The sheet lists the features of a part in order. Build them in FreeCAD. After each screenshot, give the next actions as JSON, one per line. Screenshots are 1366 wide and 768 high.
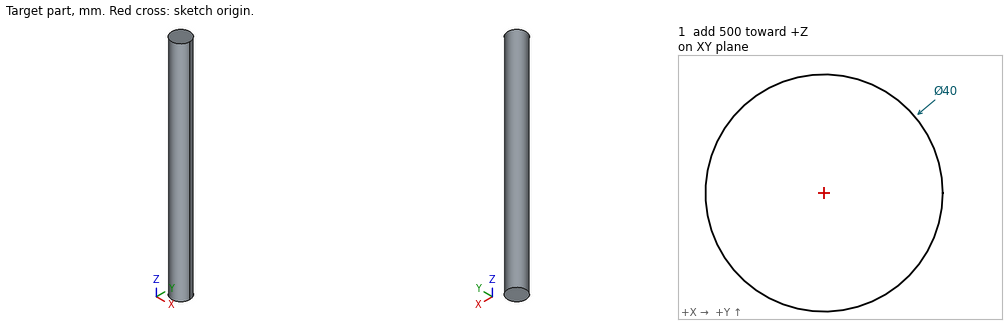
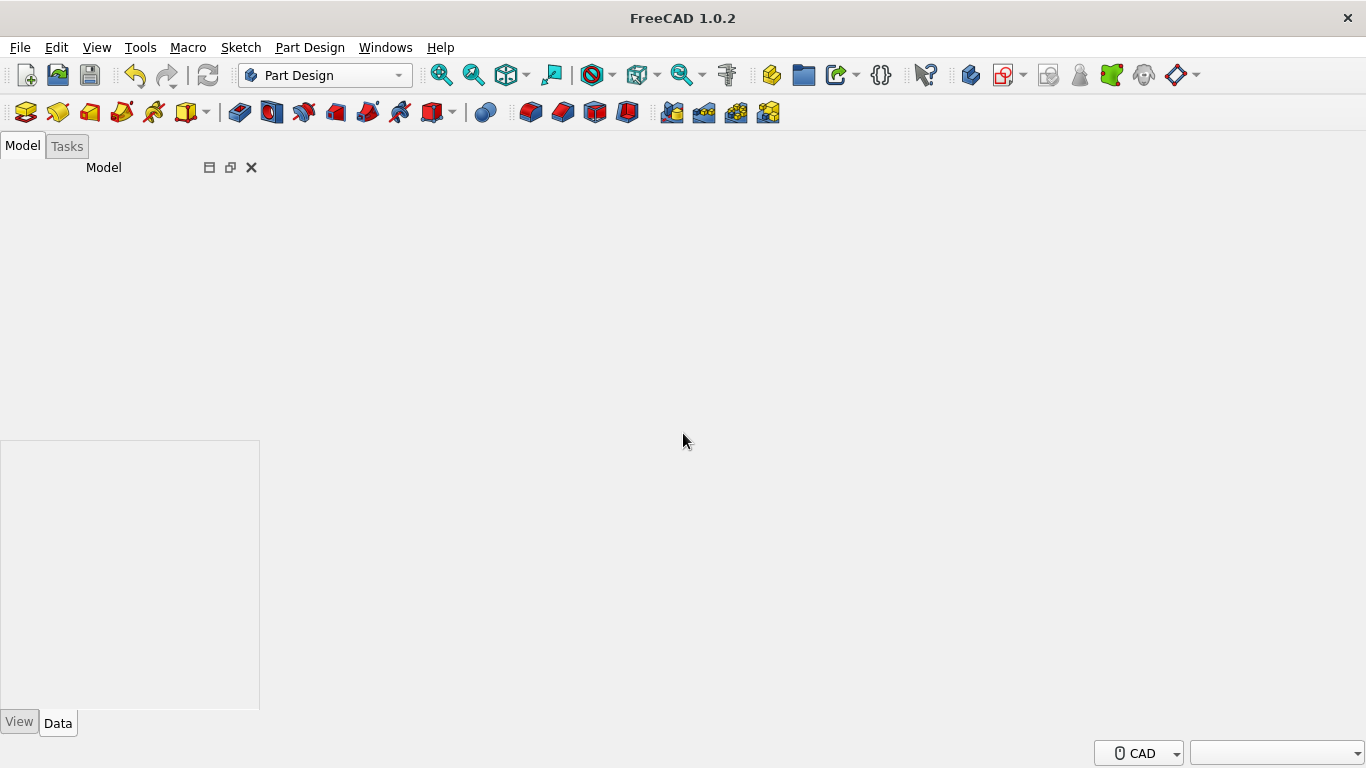
{"action": "left_click", "coordinate": [26, 76]}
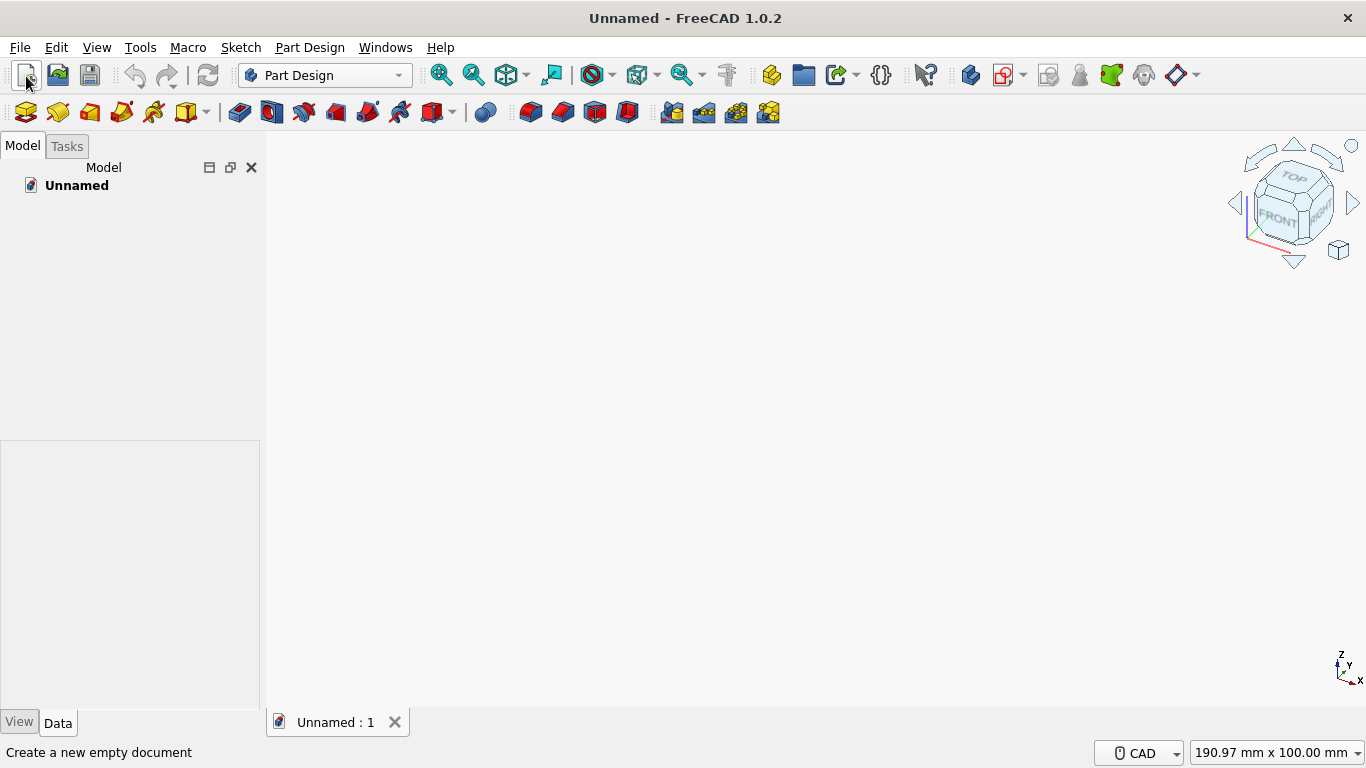
{"action": "left_click", "coordinate": [1004, 76]}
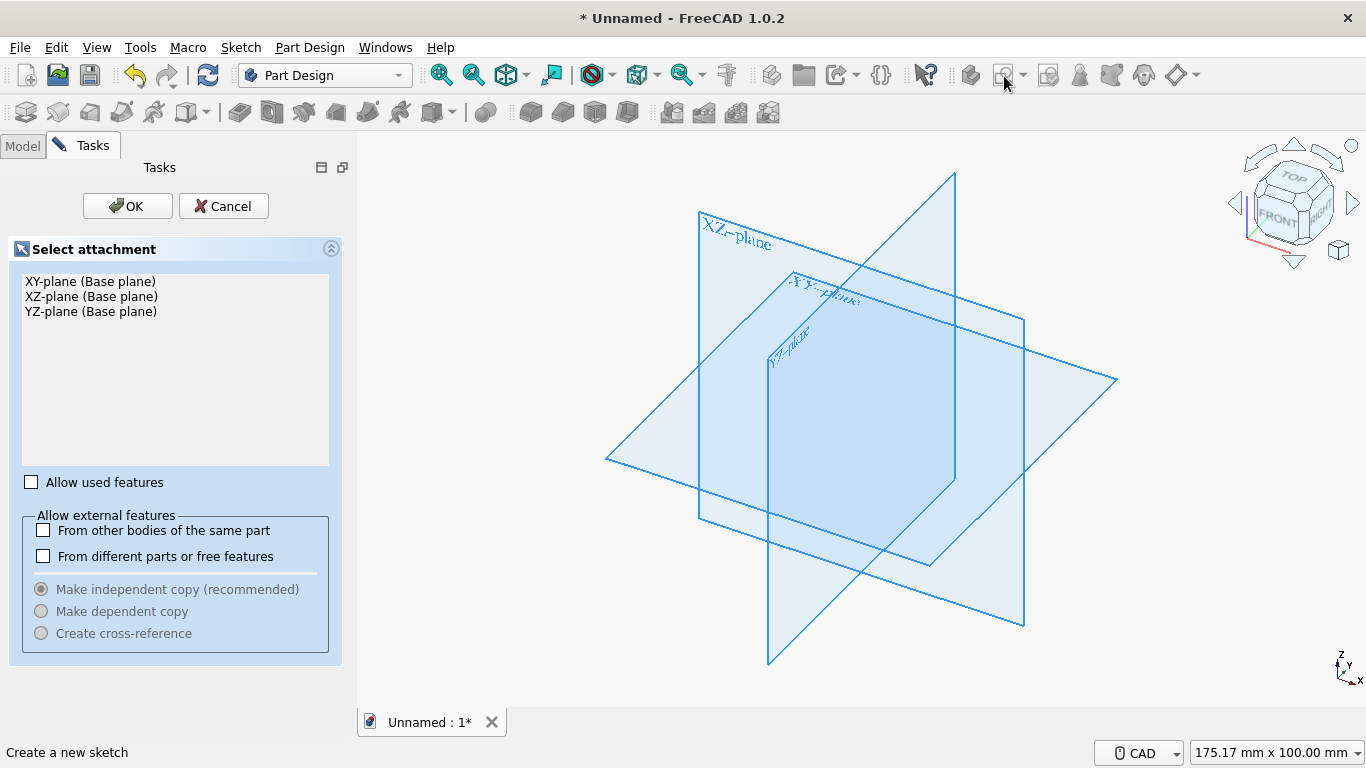
{"action": "left_click", "coordinate": [82, 282]}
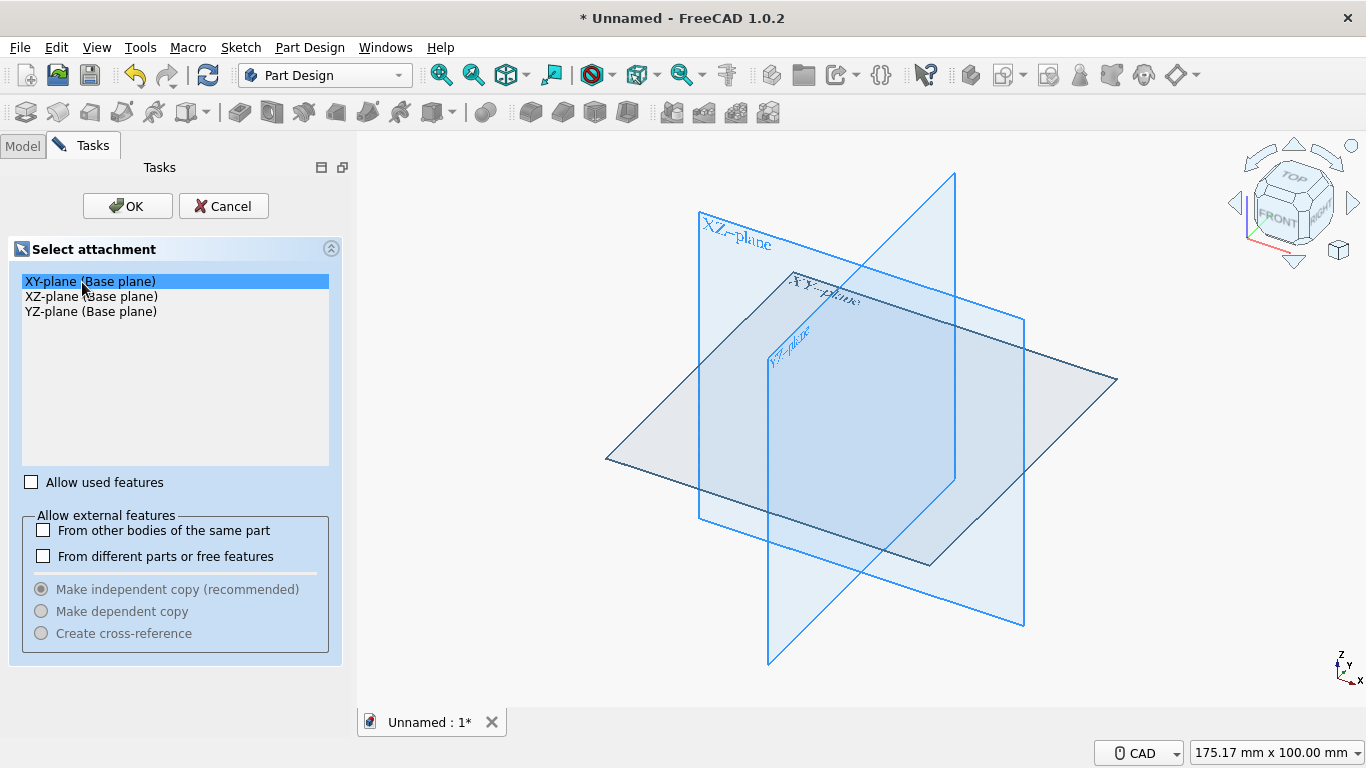
{"action": "left_click", "coordinate": [128, 206]}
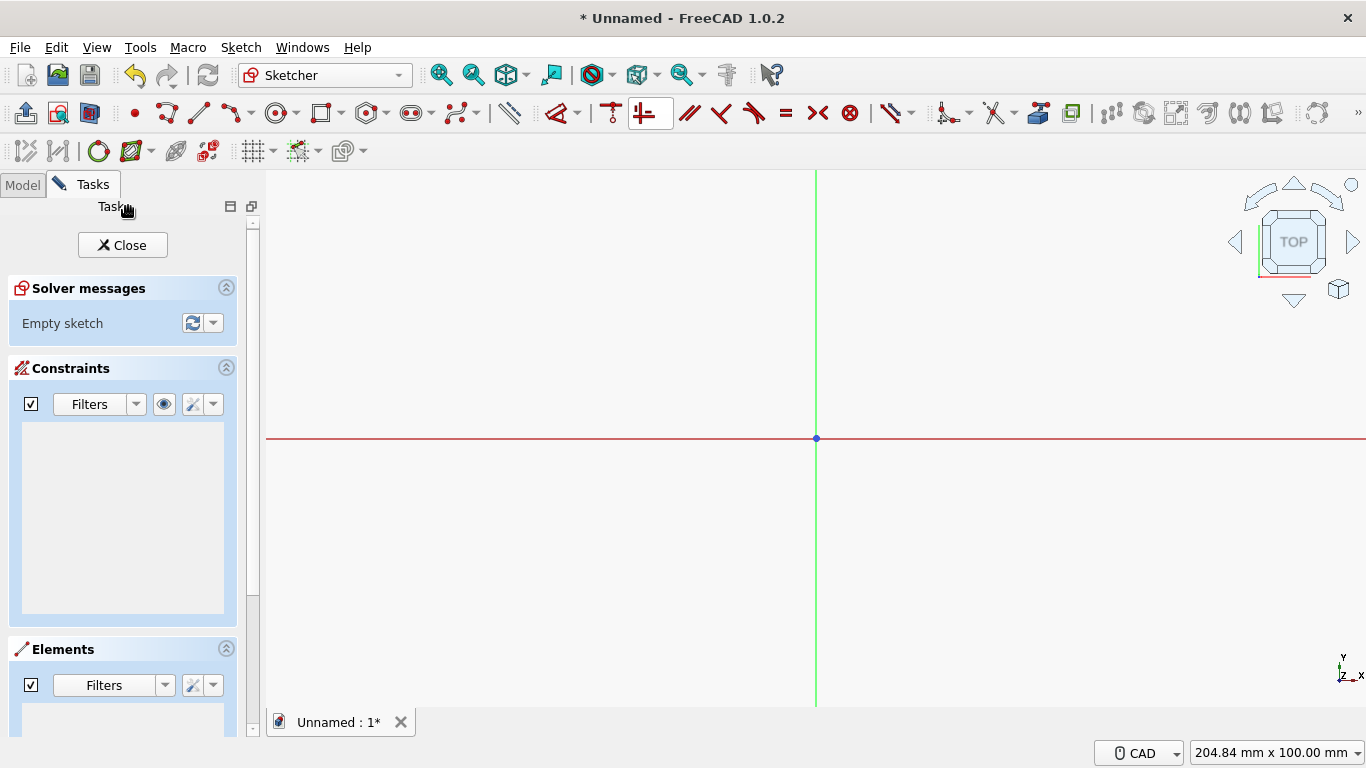
{"action": "scroll", "coordinate": [955, 439], "scroll_direction": "up", "scroll_amount": 2}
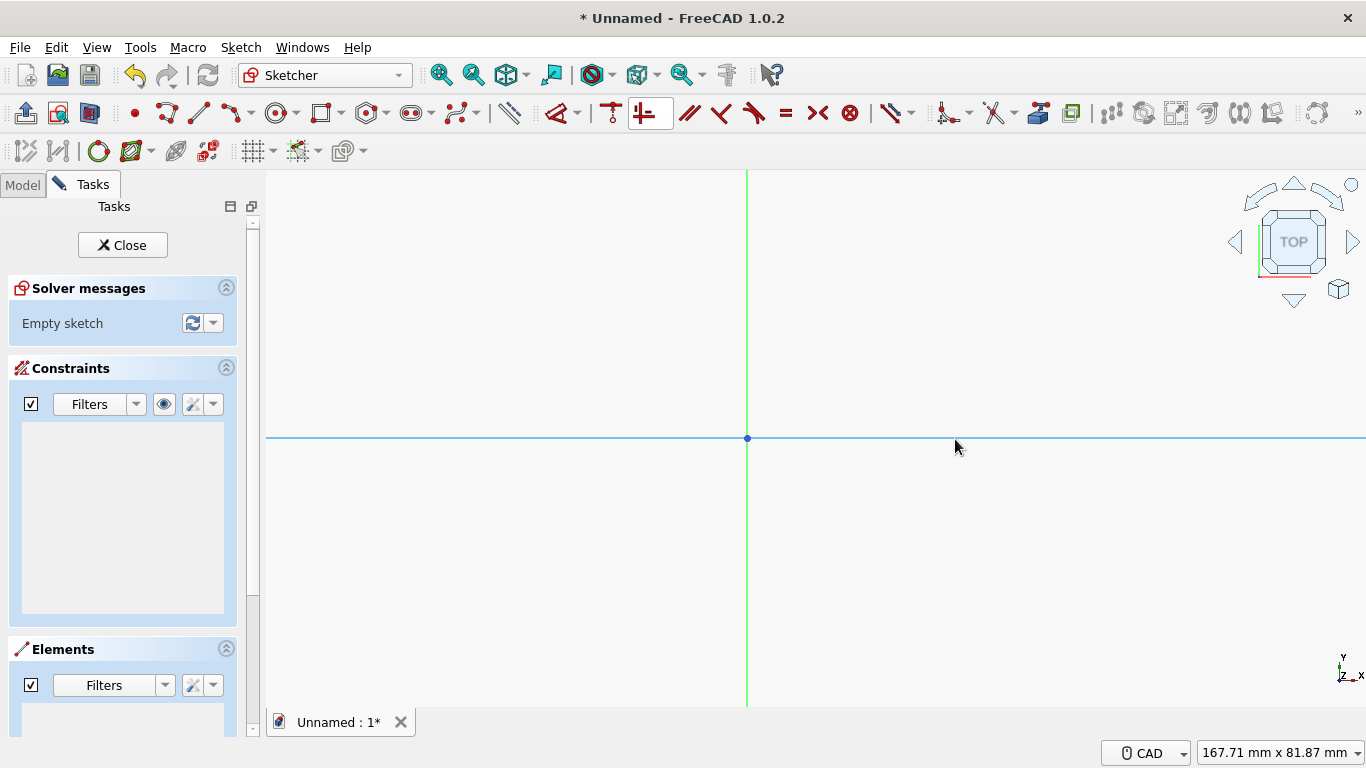
{"action": "left_click", "coordinate": [276, 114]}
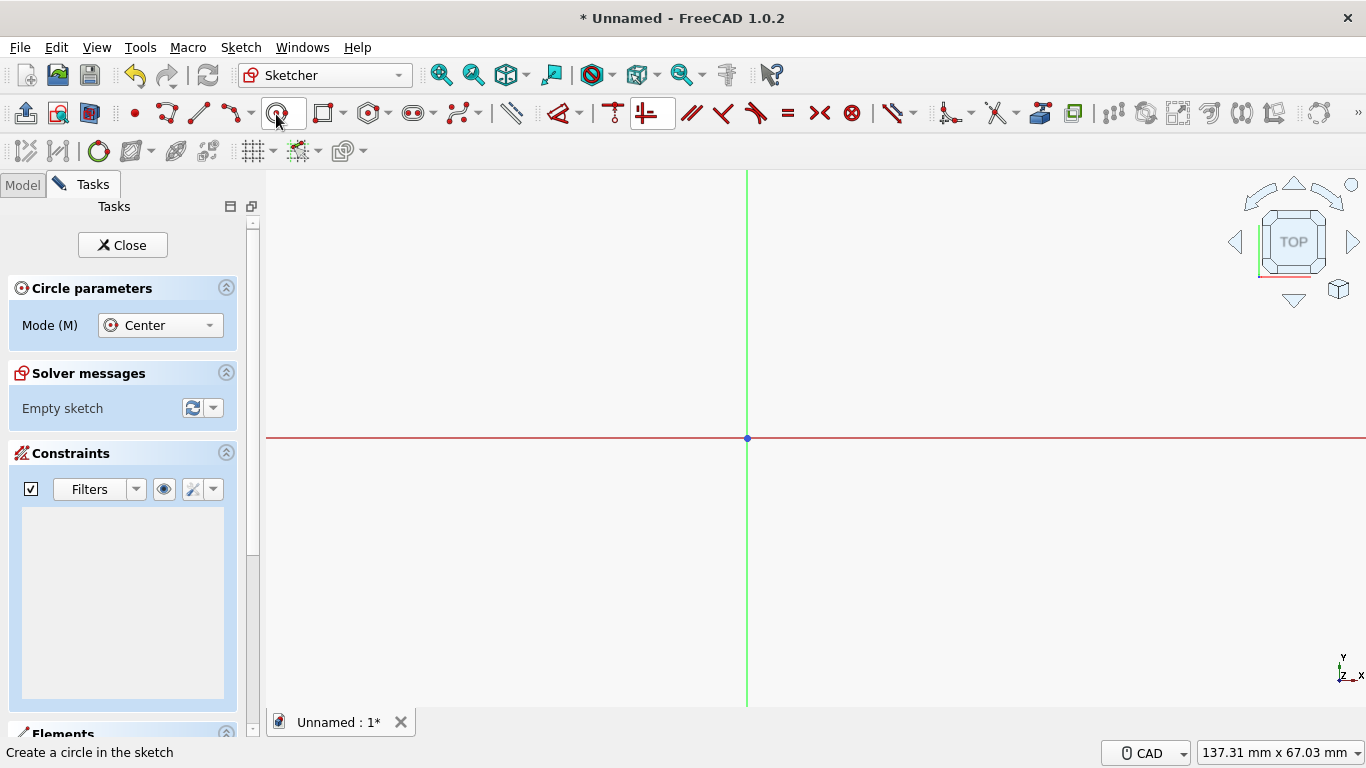
{"action": "left_click", "coordinate": [747, 438]}
{"action": "mouse_move", "coordinate": [861, 325]}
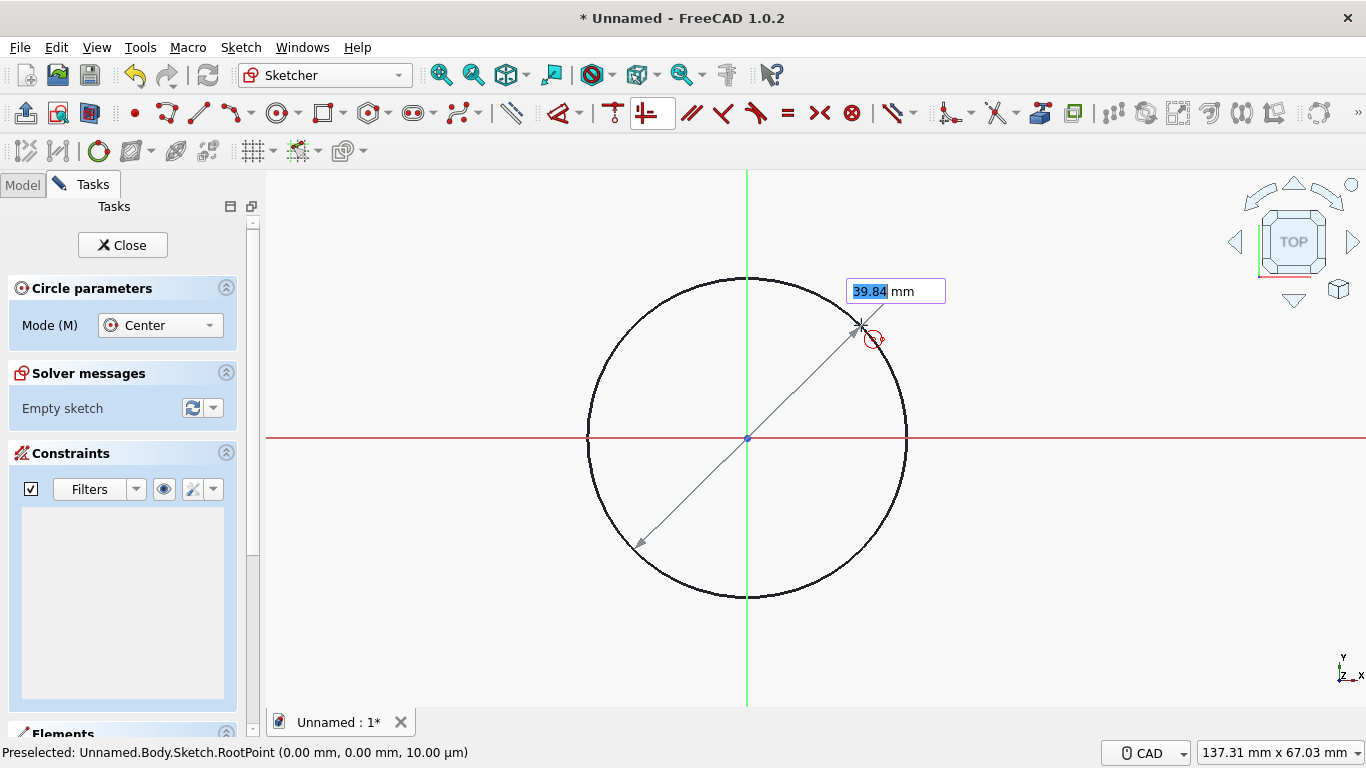
{"action": "type", "text": "40"}
{"action": "key", "text": "Return"}
{"action": "key", "text": "Escape"}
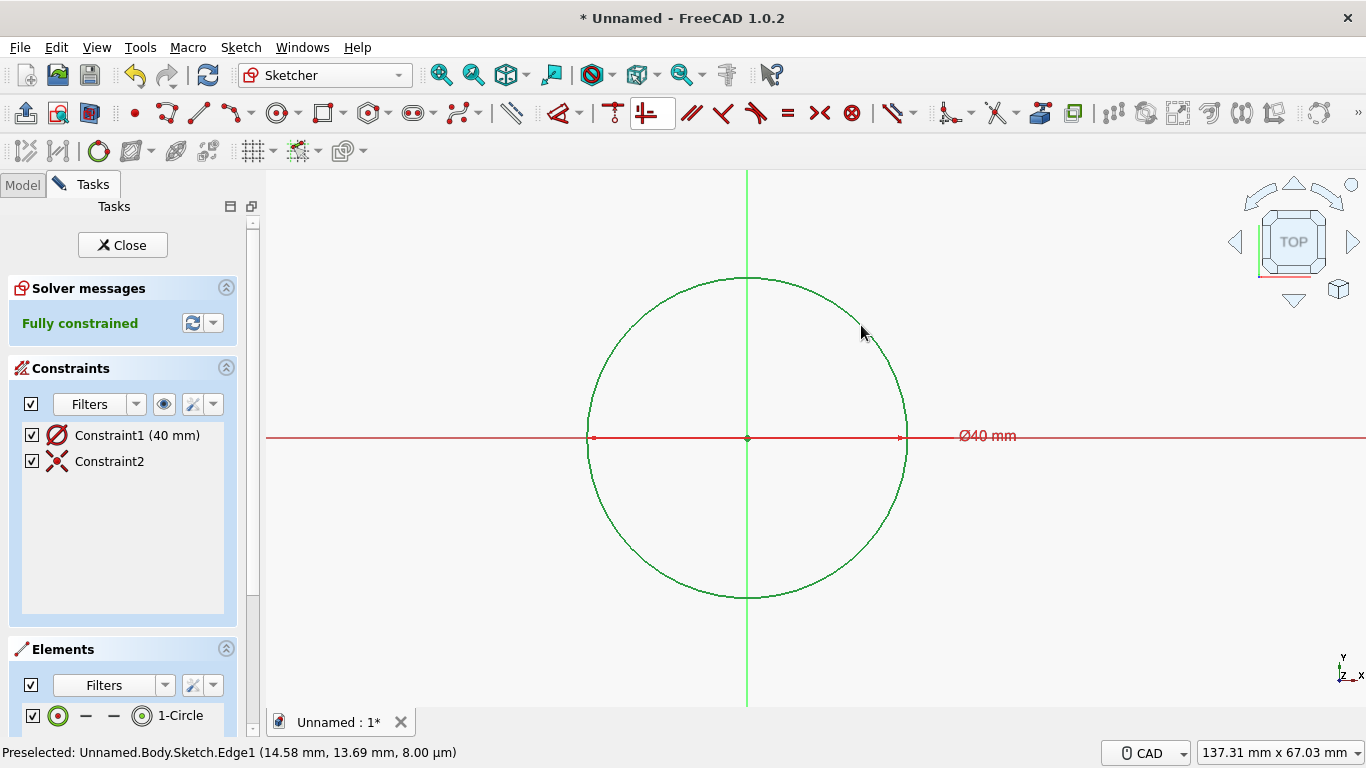
{"action": "left_click", "coordinate": [123, 245]}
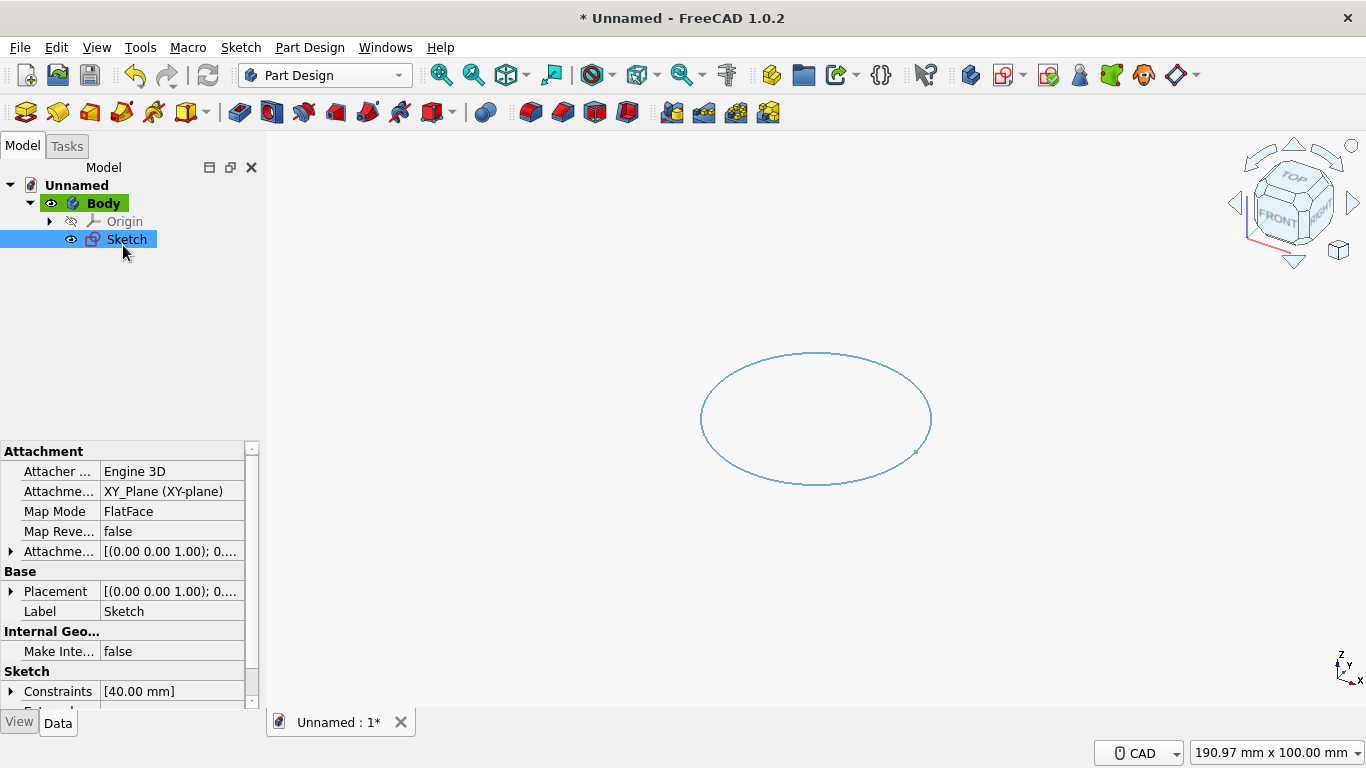
{"action": "left_click", "coordinate": [26, 112]}